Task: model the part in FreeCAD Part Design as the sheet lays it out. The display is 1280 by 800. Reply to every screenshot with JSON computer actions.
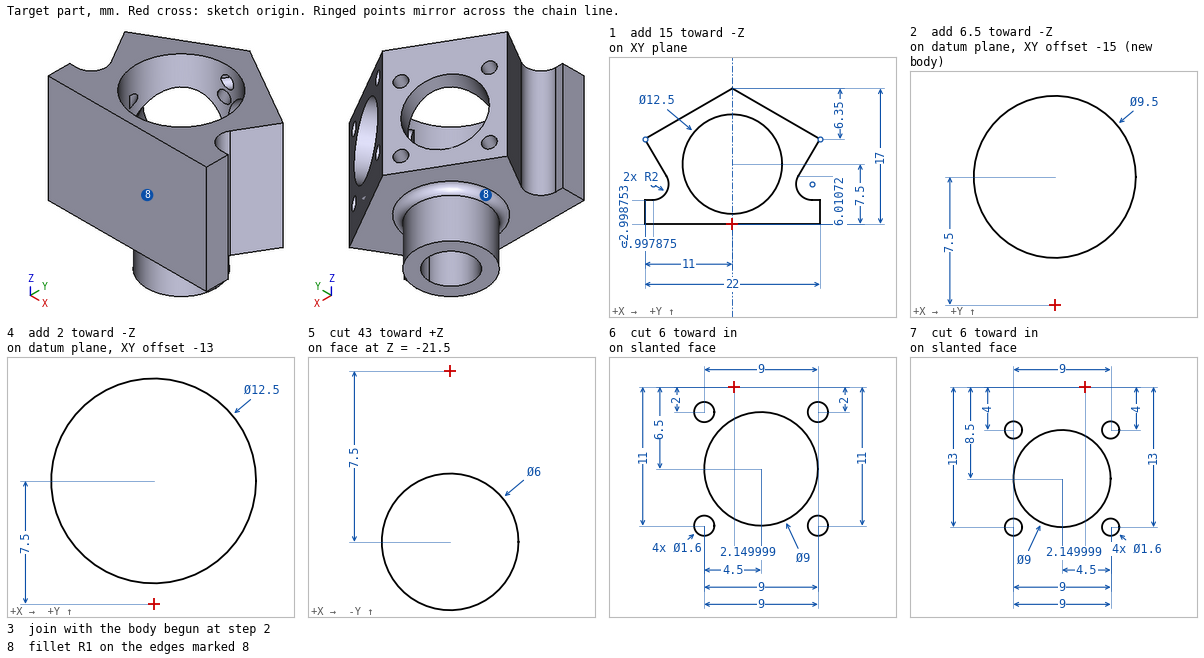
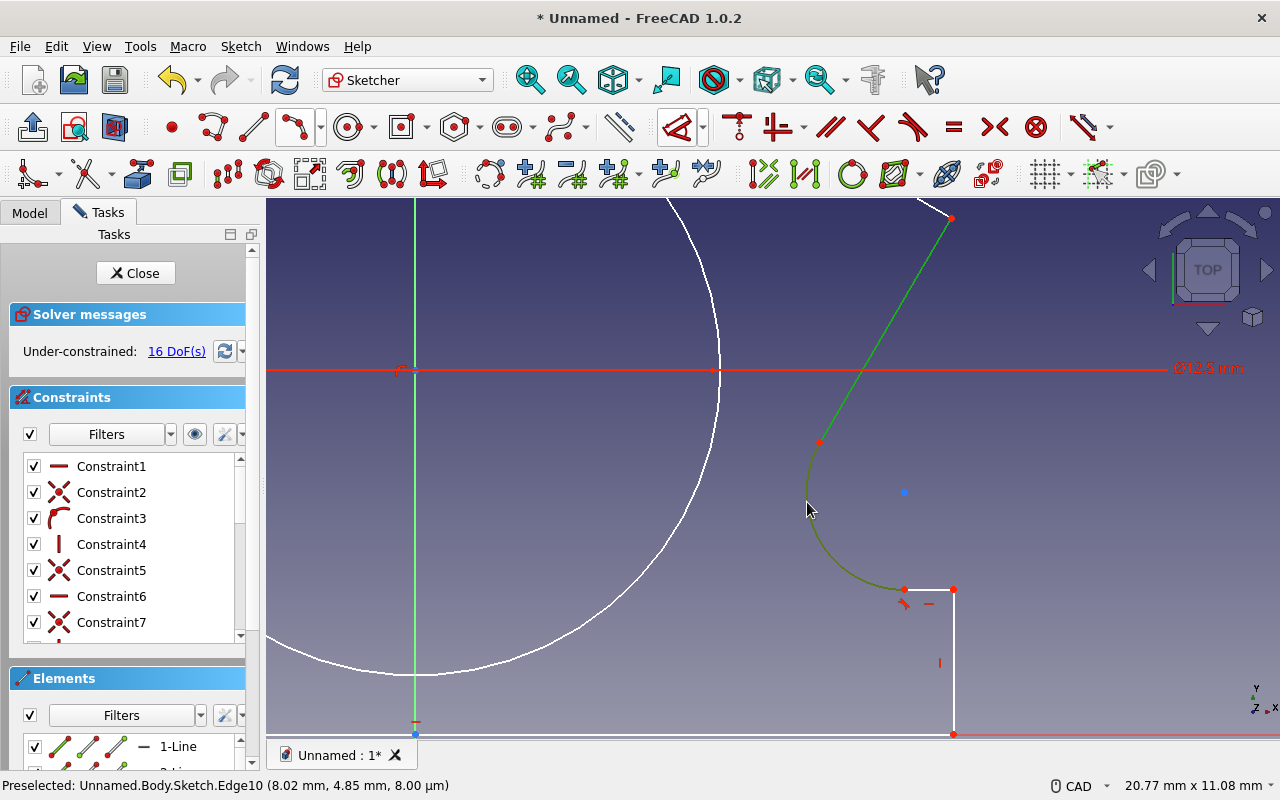
{"action": "left_click", "coordinate": [913, 128]}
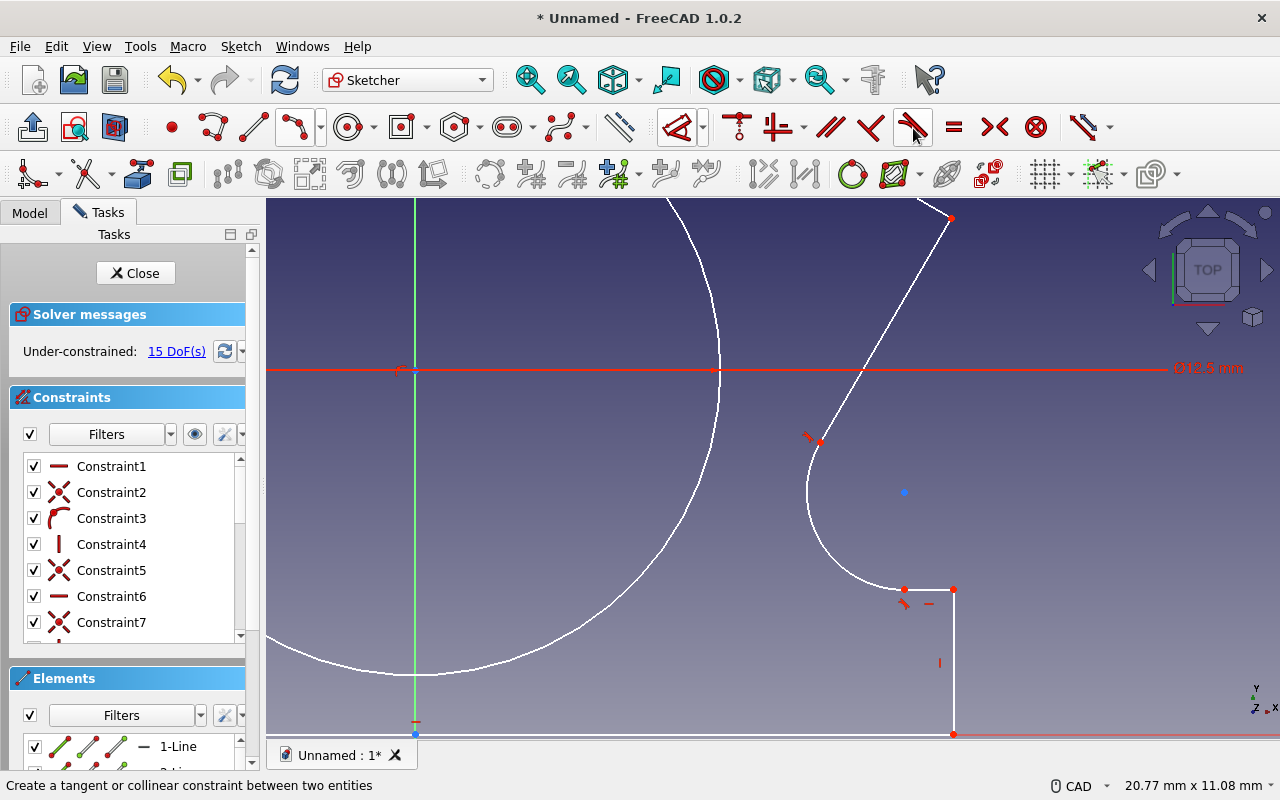
{"action": "scroll", "coordinate": [940, 590], "scroll_direction": "down", "scroll_amount": 4}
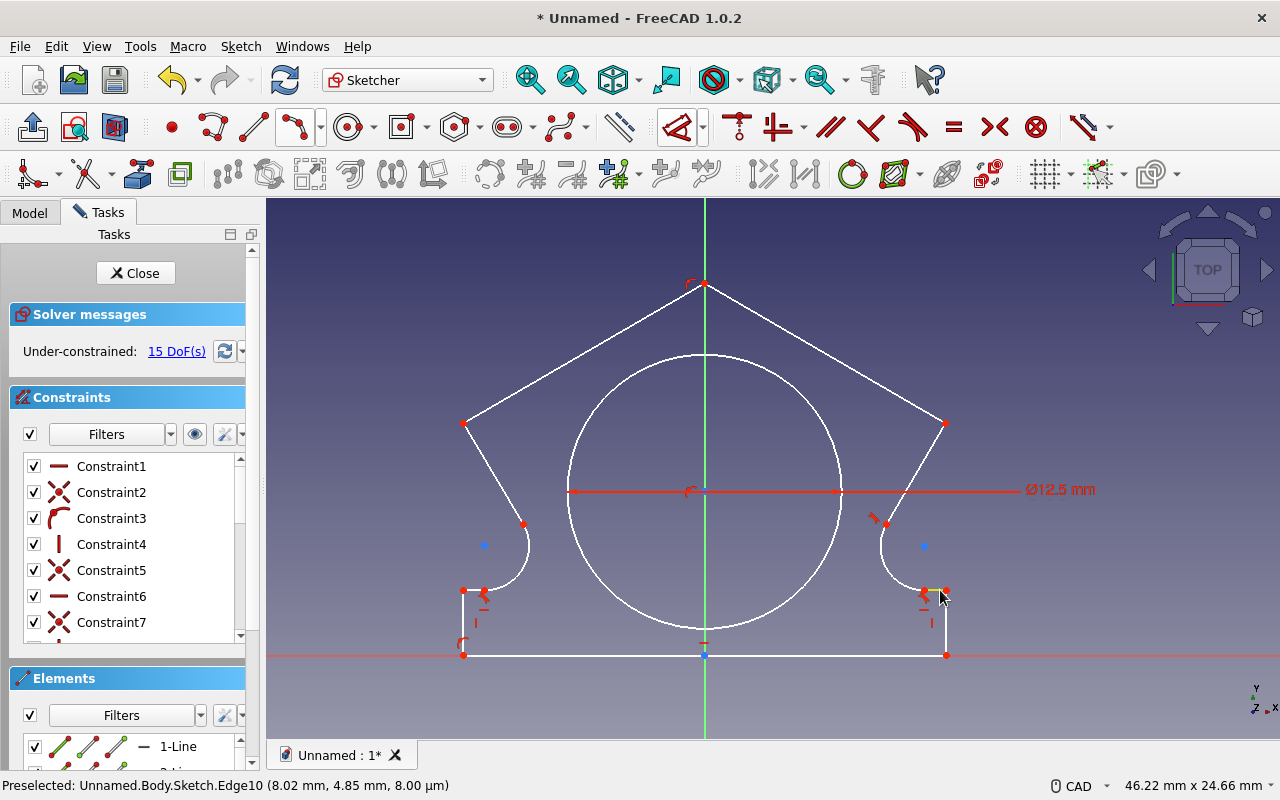
{"action": "left_click", "coordinate": [481, 454]}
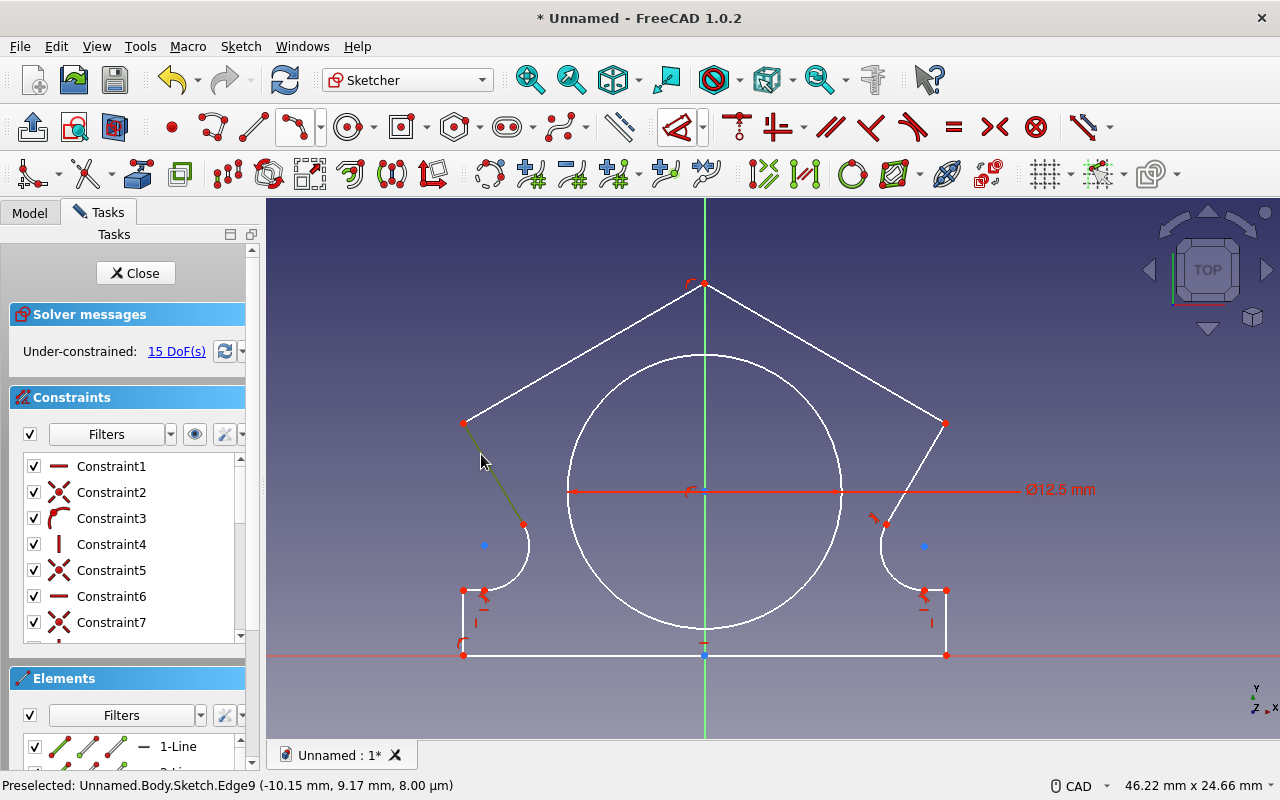
{"action": "left_click", "coordinate": [511, 582]}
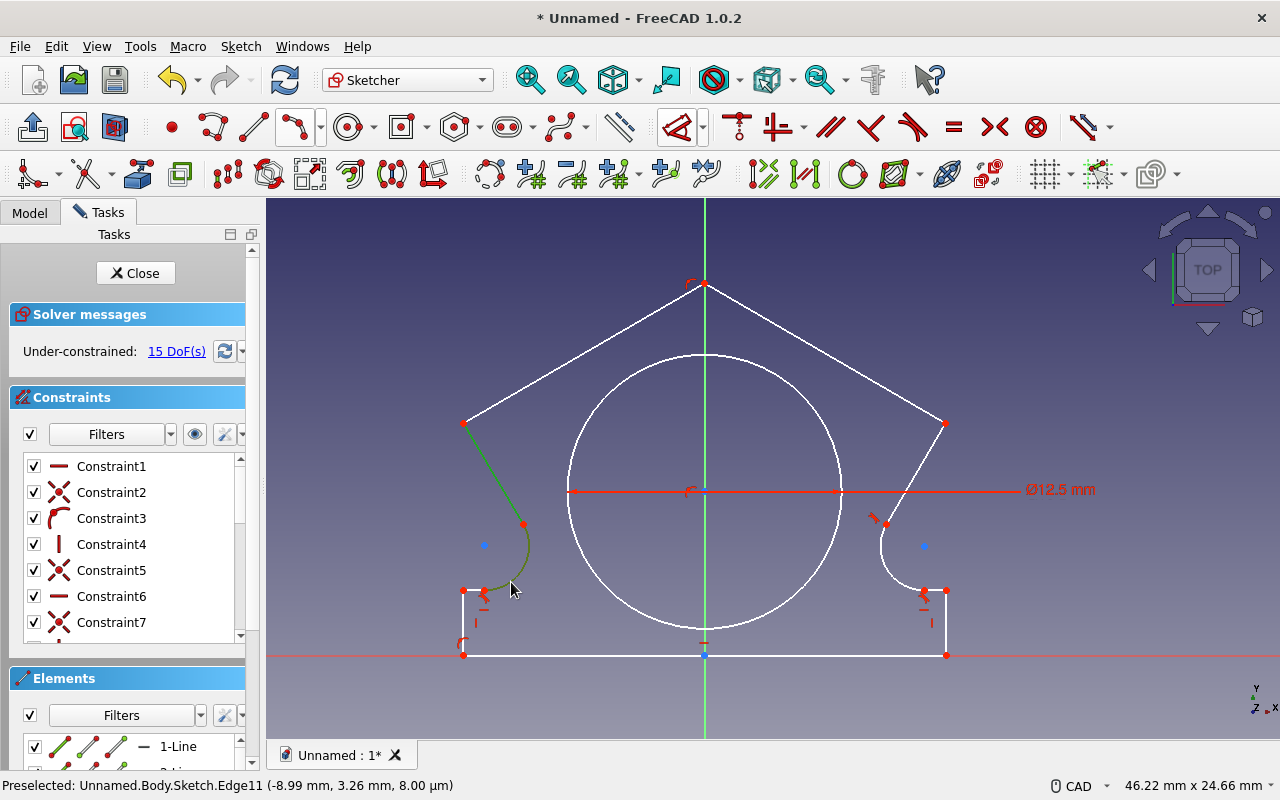
{"action": "left_click", "coordinate": [913, 128]}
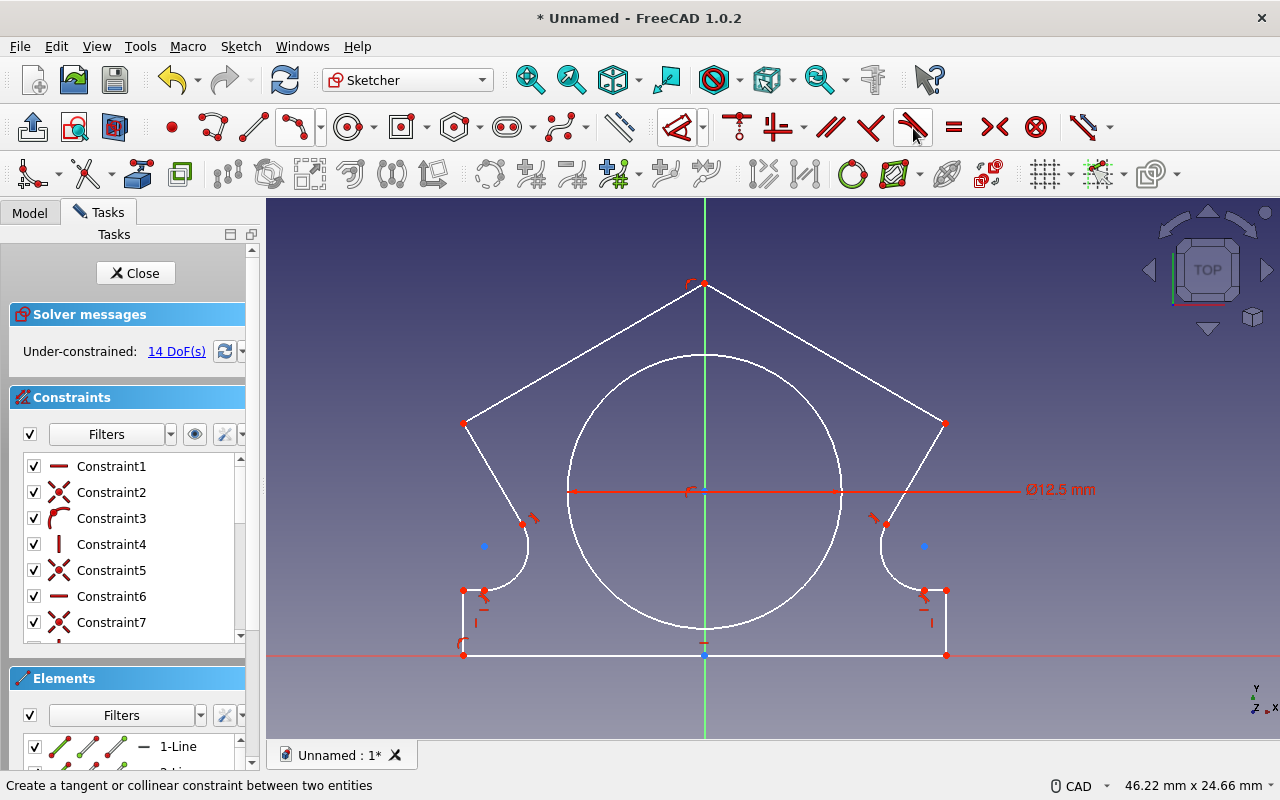
{"action": "left_click", "coordinate": [881, 551]}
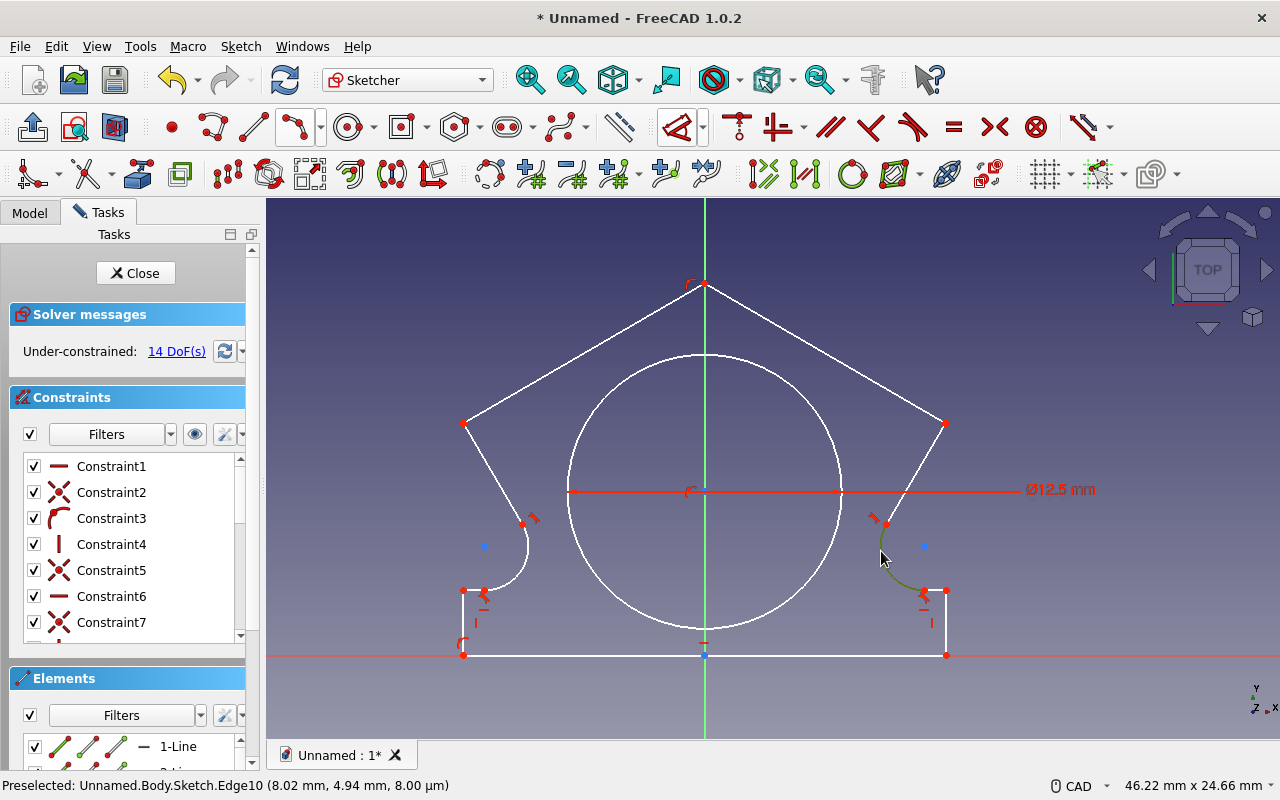
{"action": "left_click", "coordinate": [510, 582]}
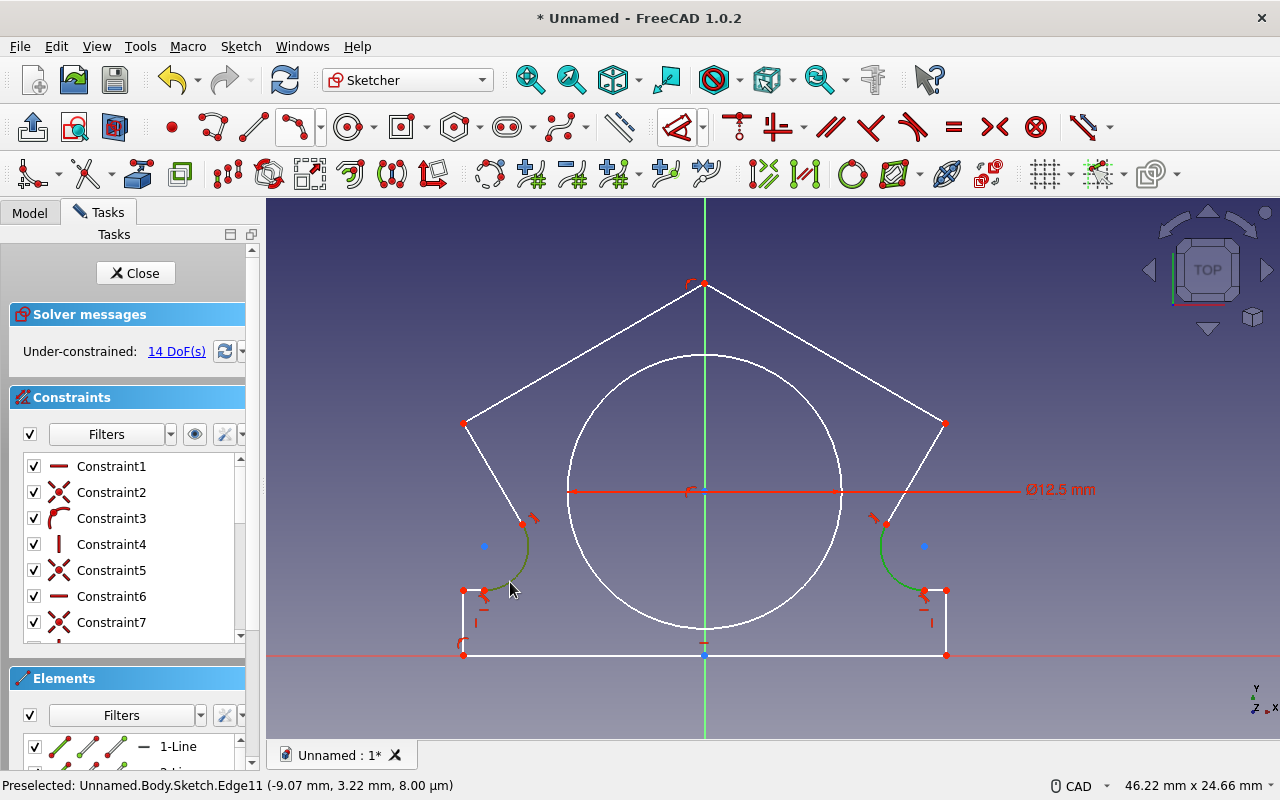
{"action": "left_click", "coordinate": [954, 128]}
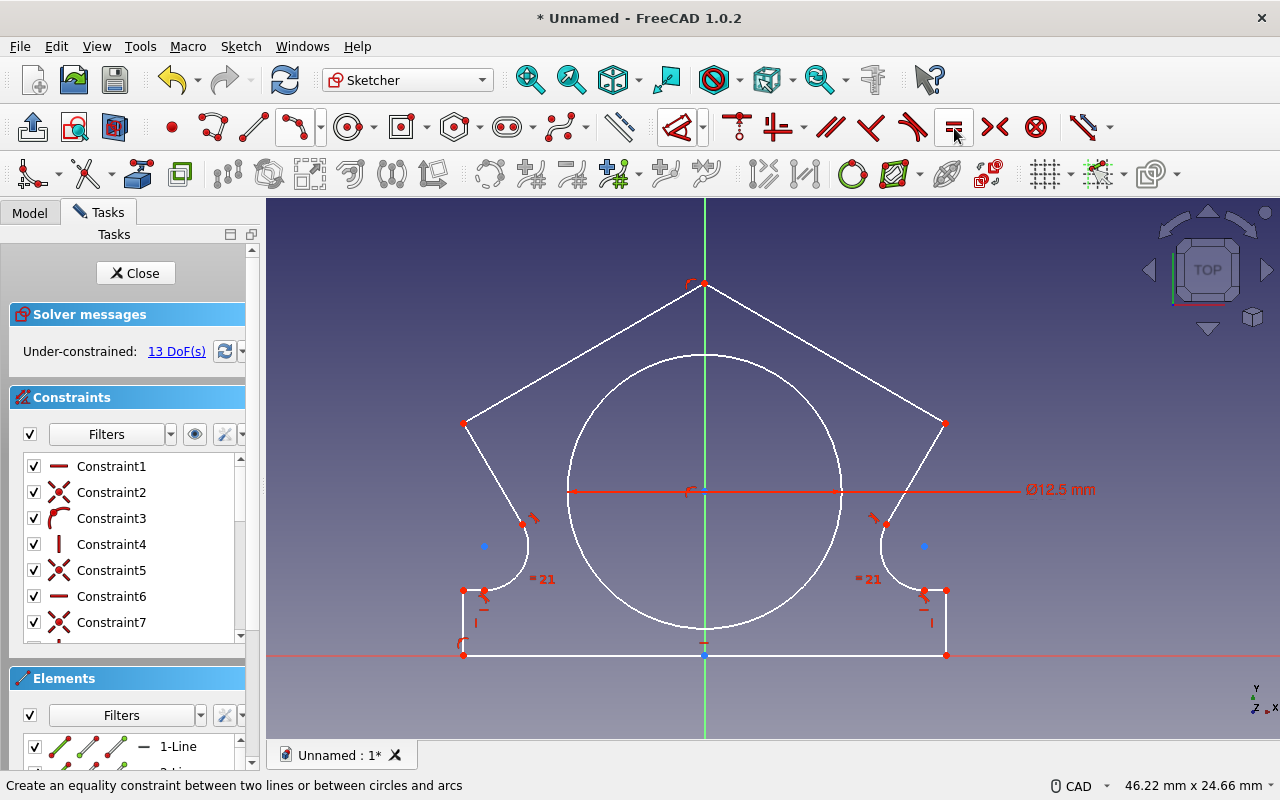
{"action": "left_click", "coordinate": [924, 546]}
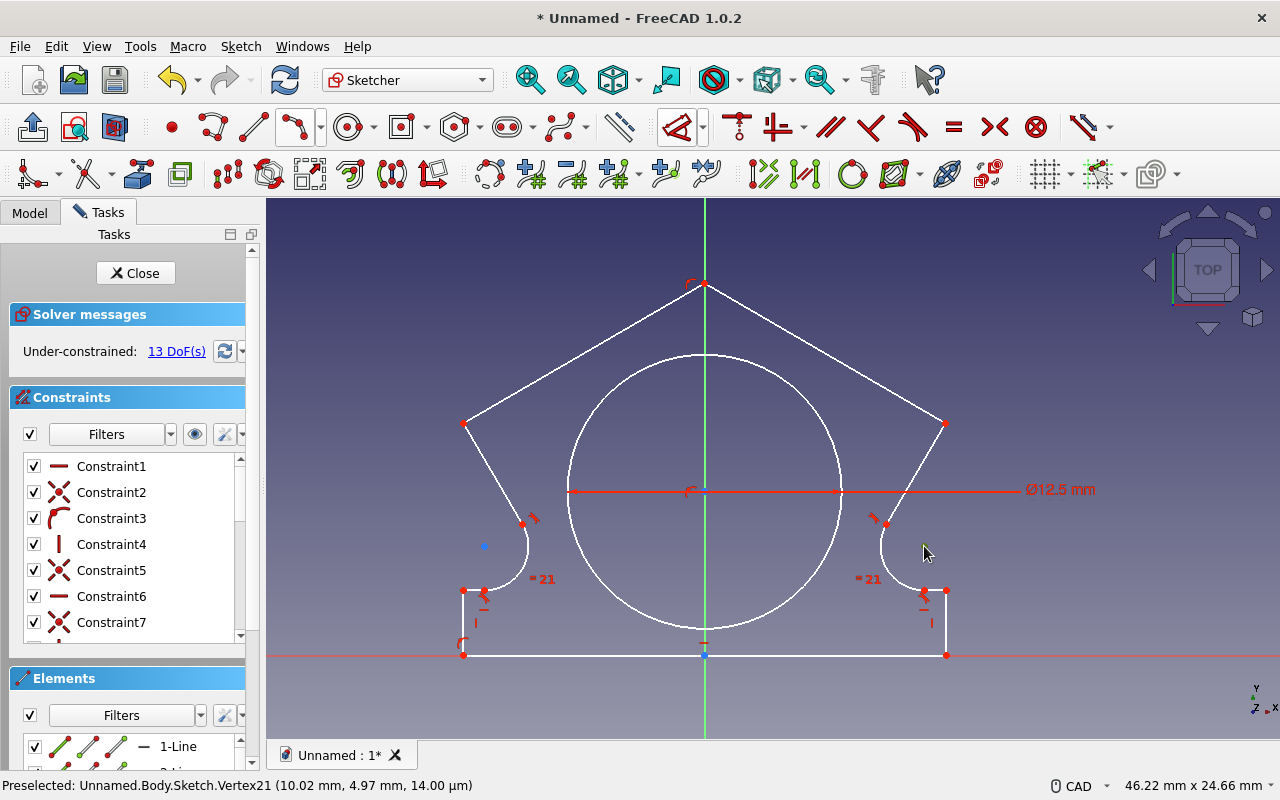
{"action": "left_click", "coordinate": [485, 546]}